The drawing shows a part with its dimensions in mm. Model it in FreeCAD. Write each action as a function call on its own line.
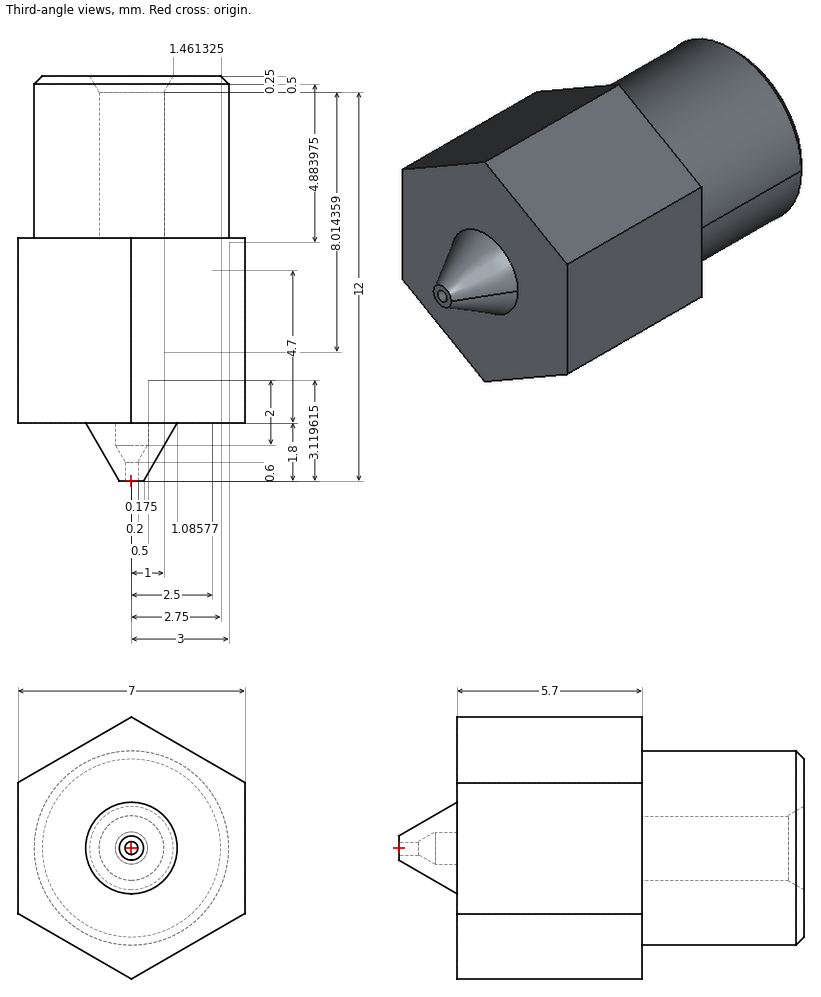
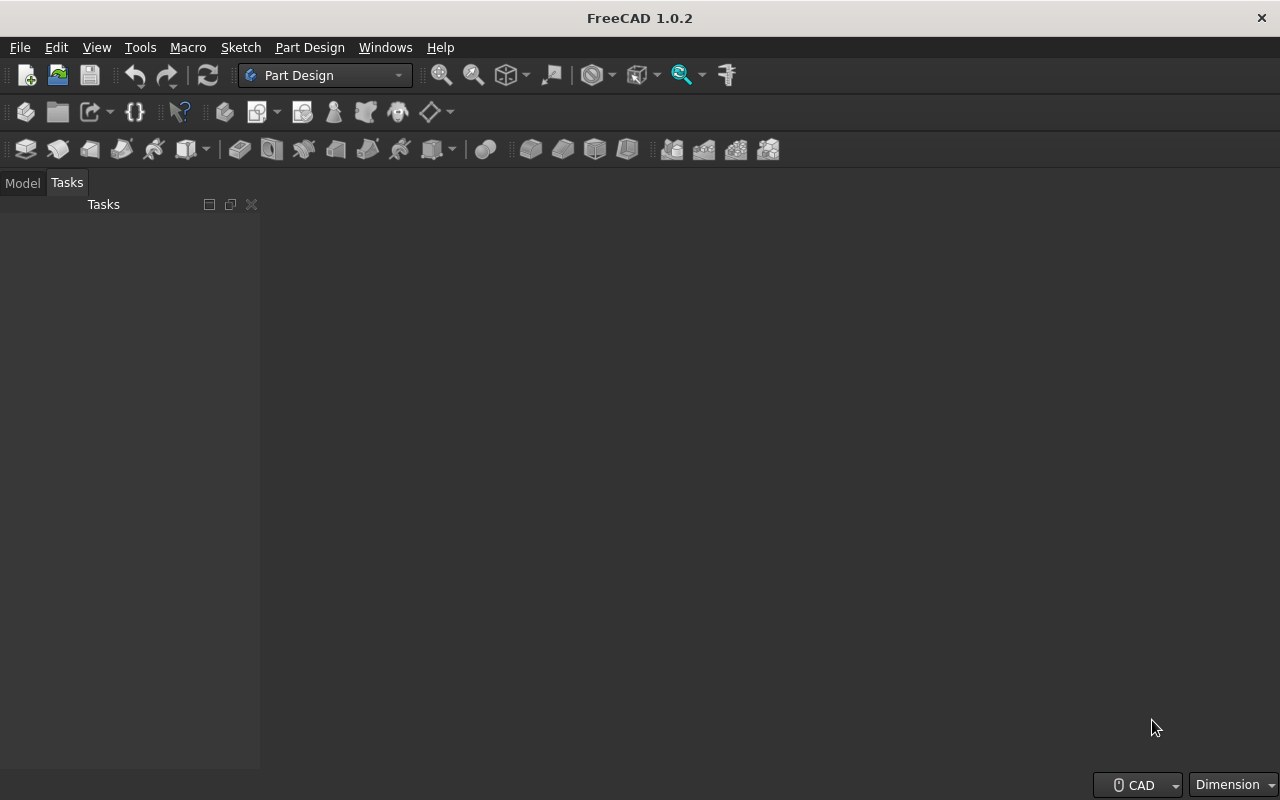
click(26, 76)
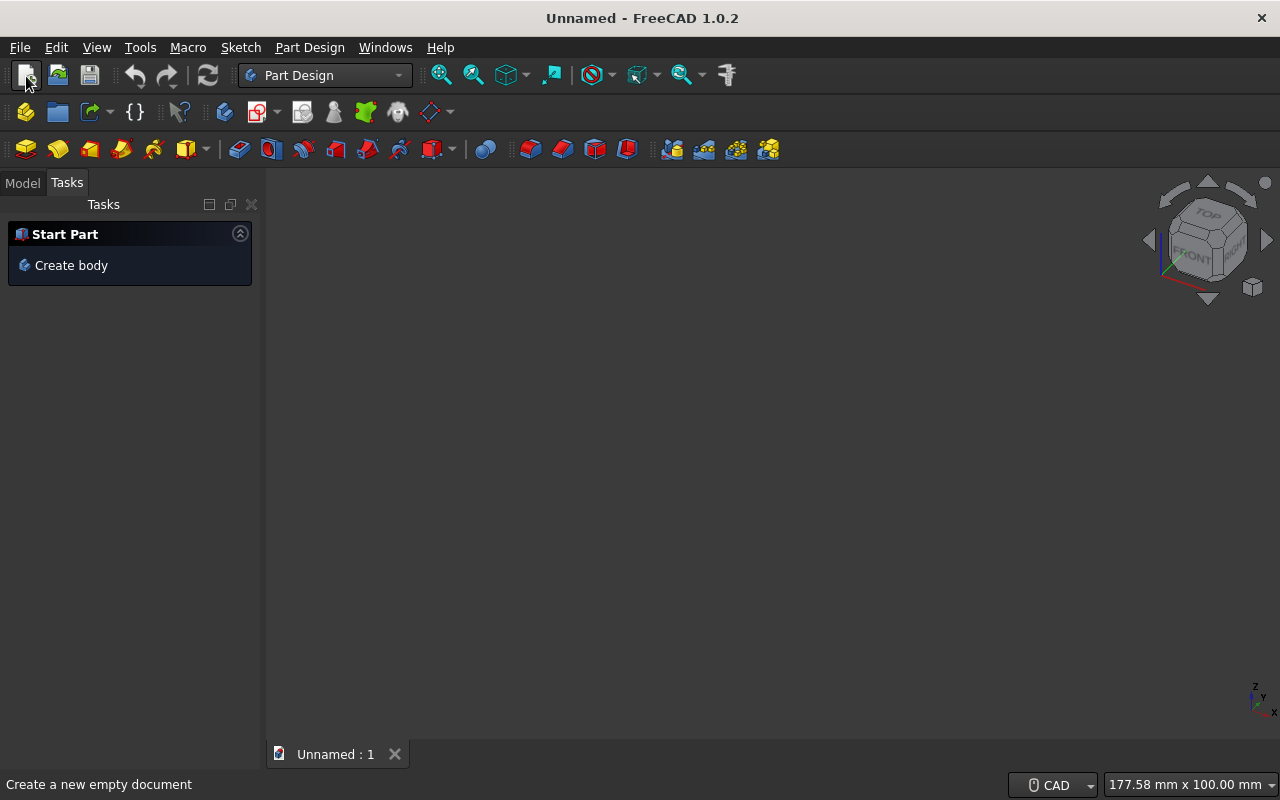
click(258, 112)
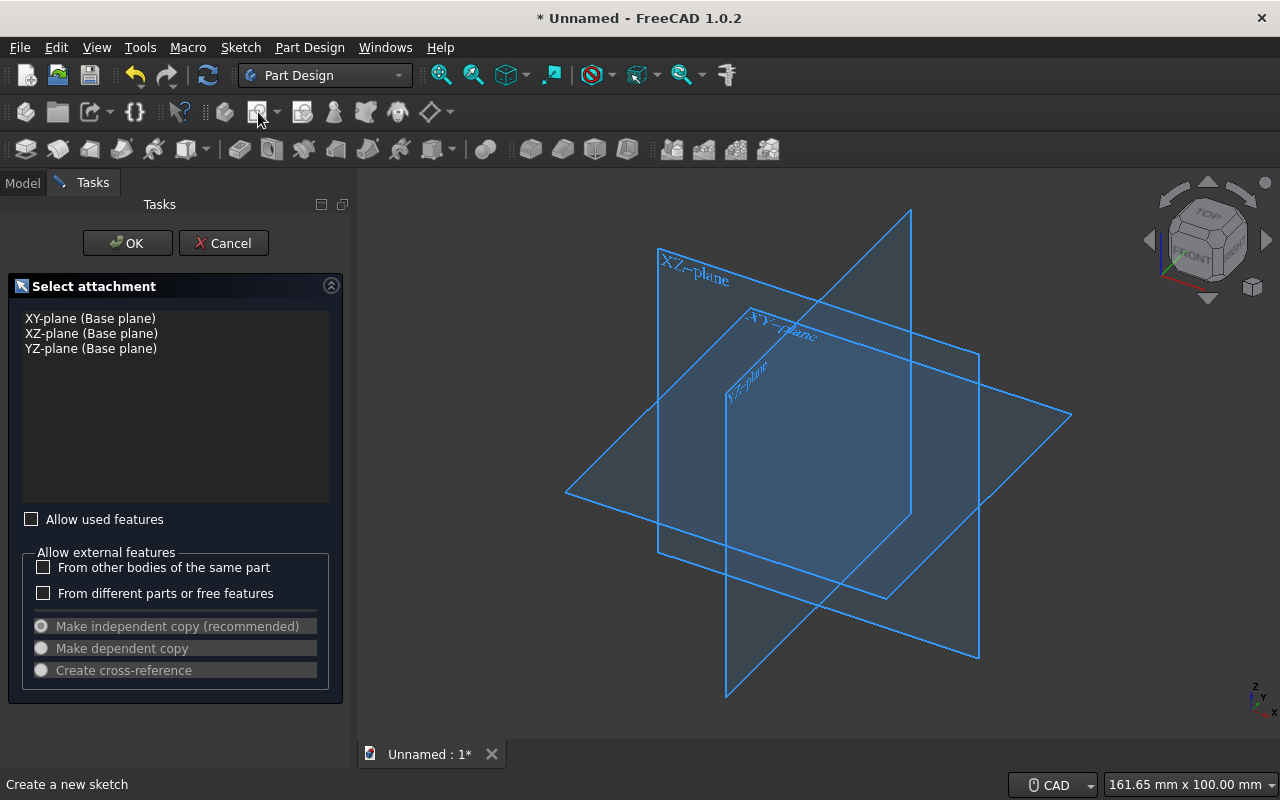
click(82, 318)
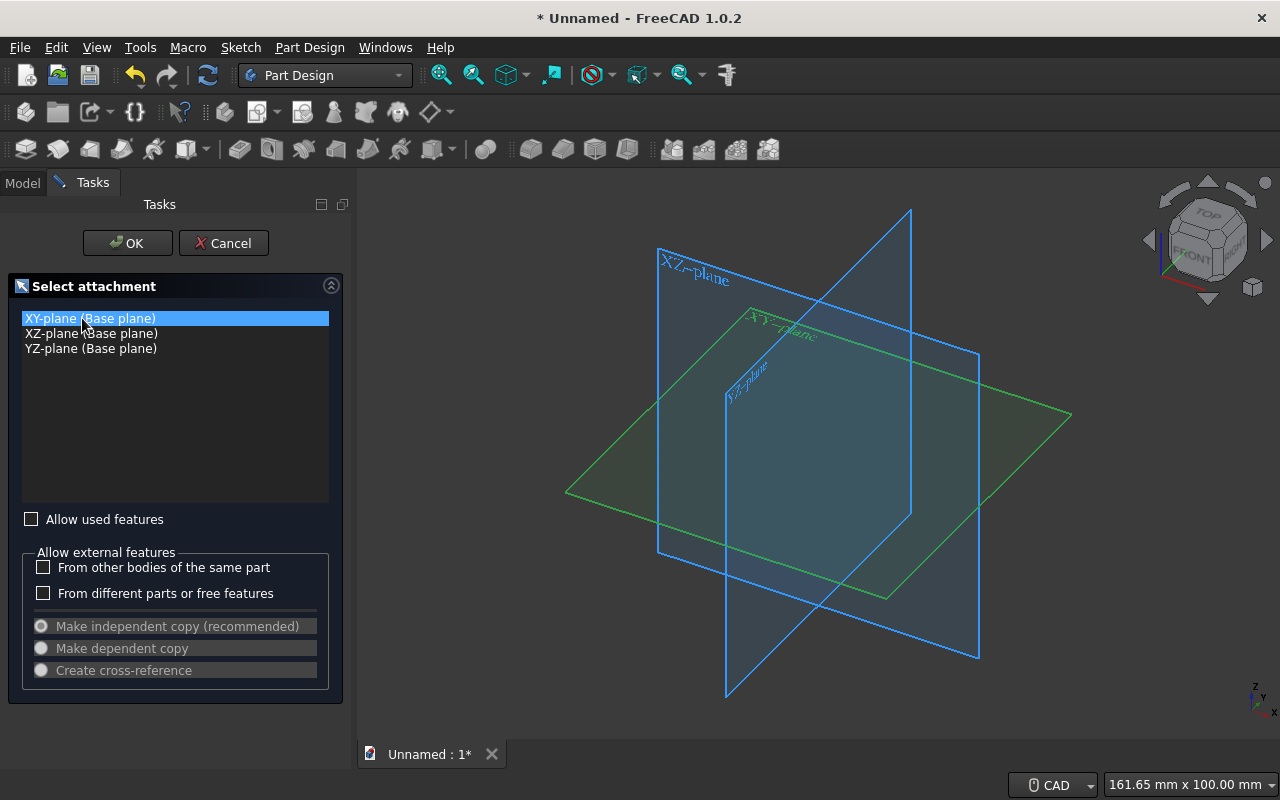
click(128, 243)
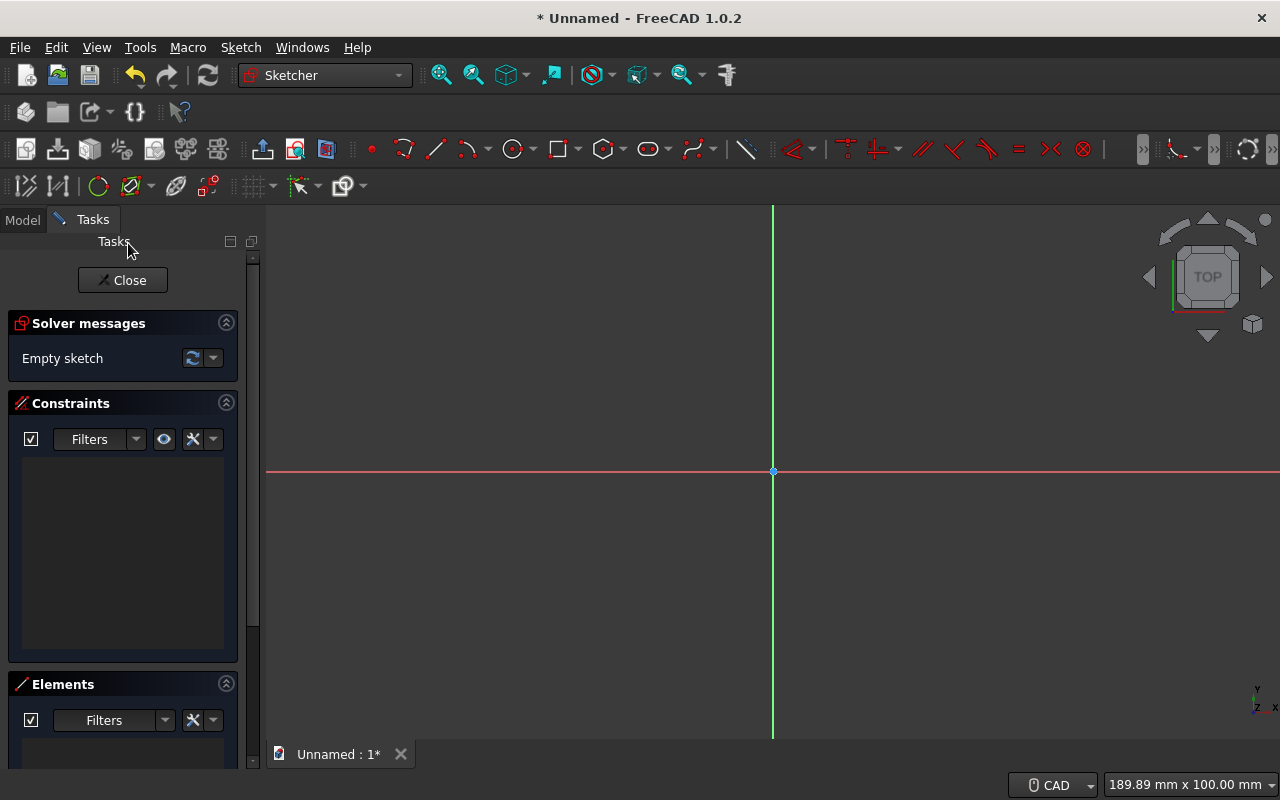
scroll(800, 430, up, 8)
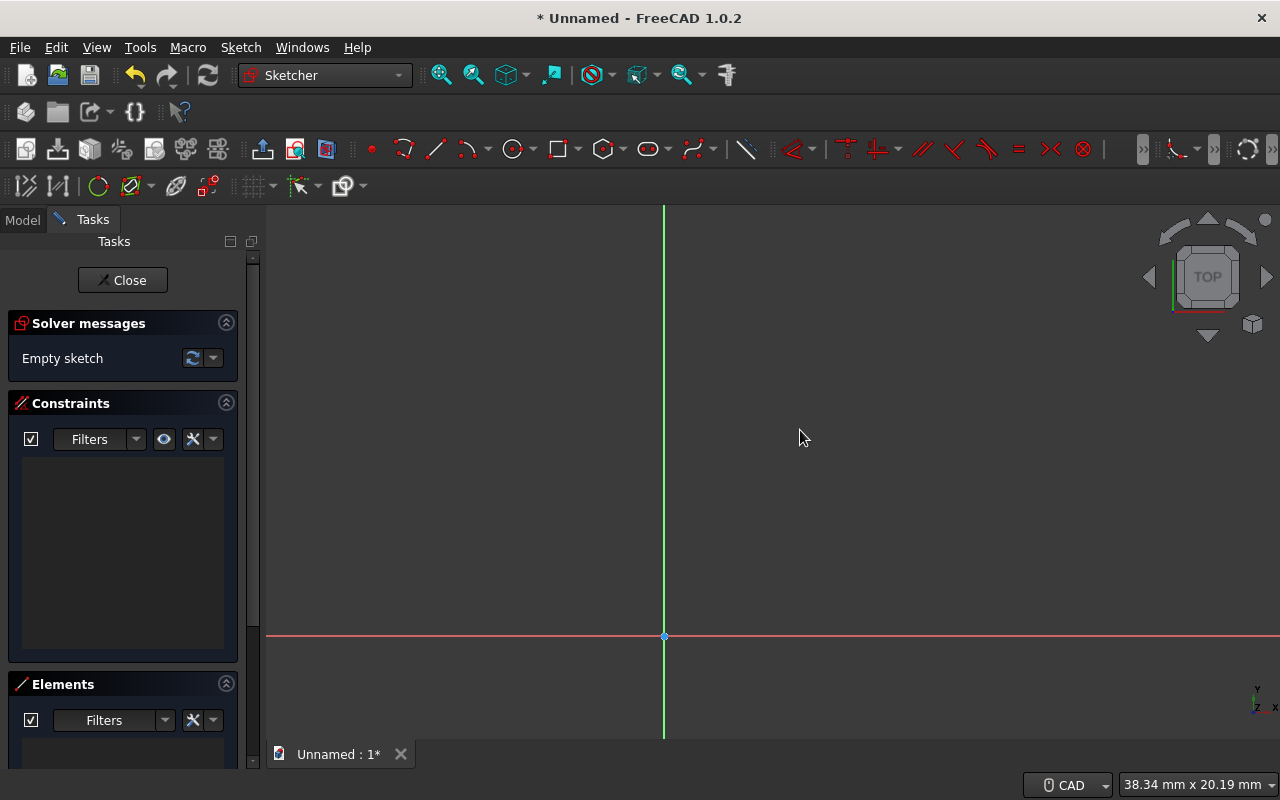
click(404, 150)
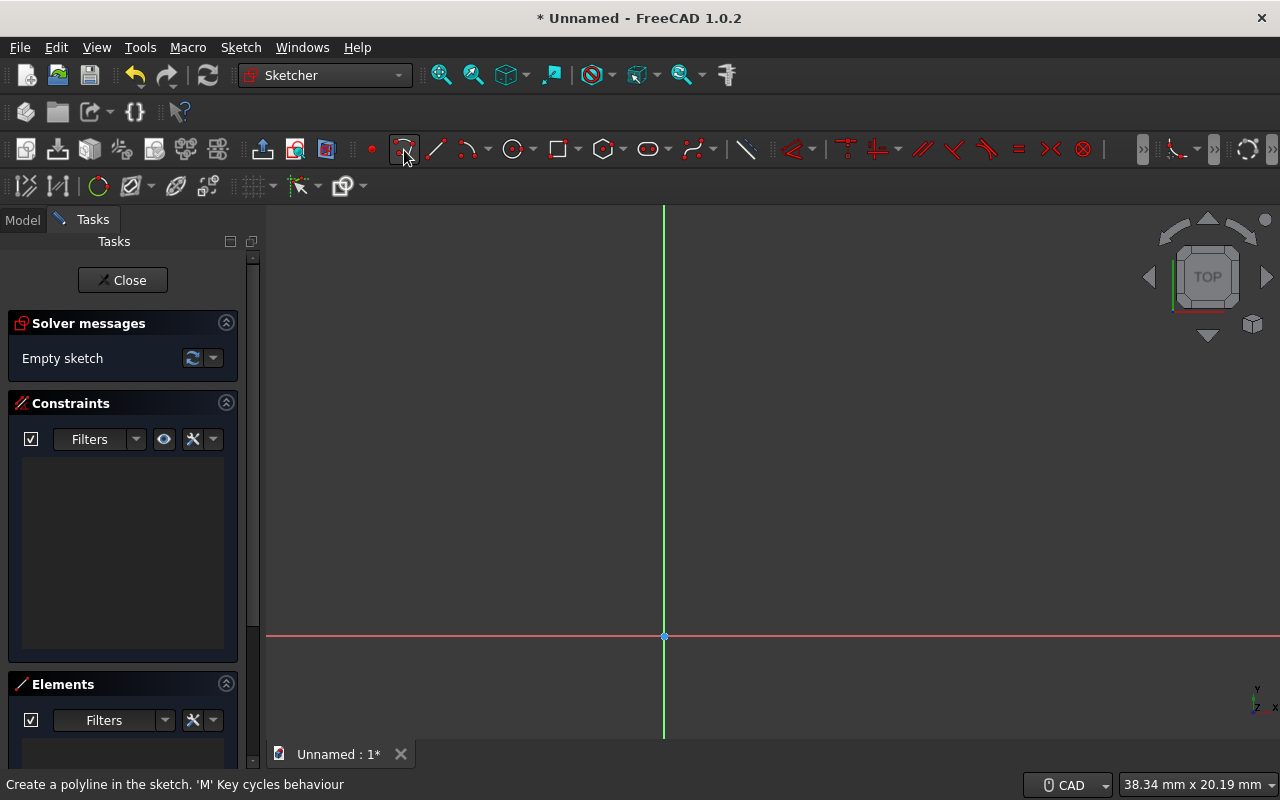
scroll(669, 636, up, 6)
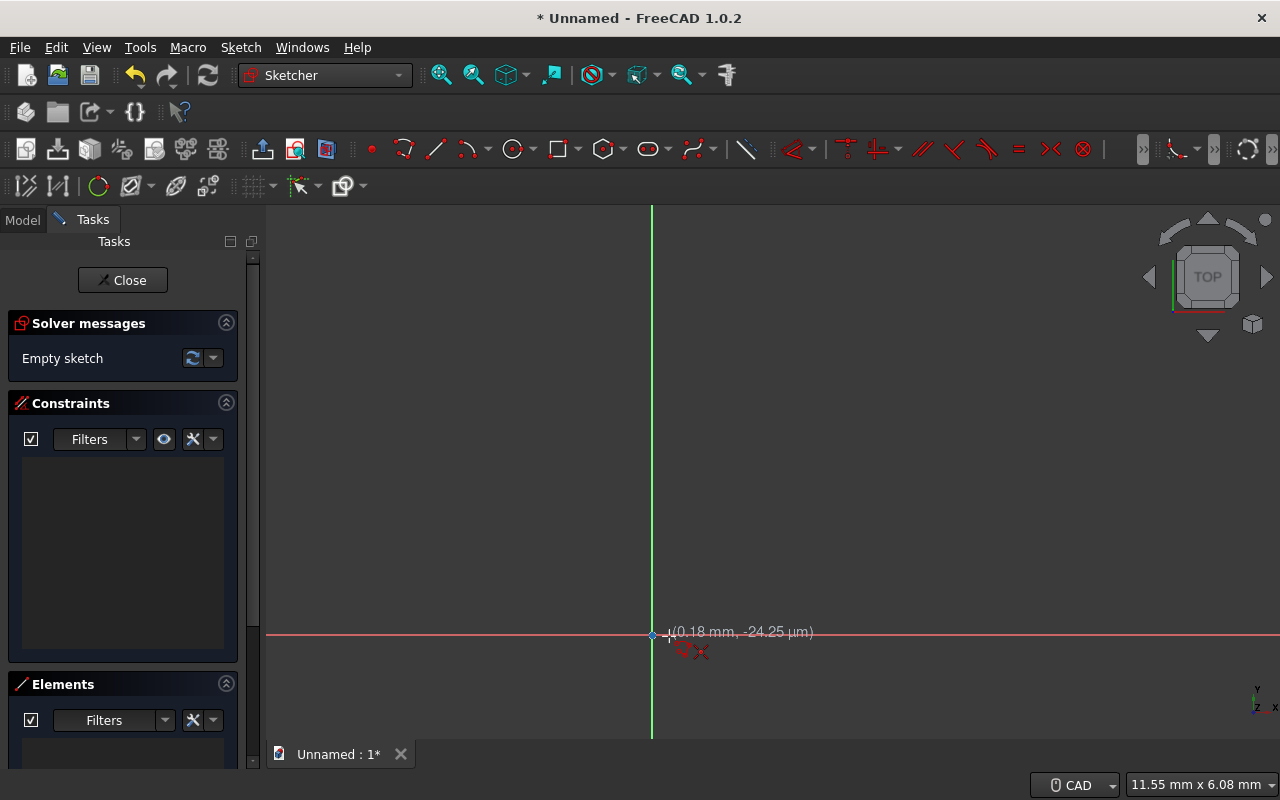
click(670, 635)
click(685, 626)
click(776, 477)
click(872, 477)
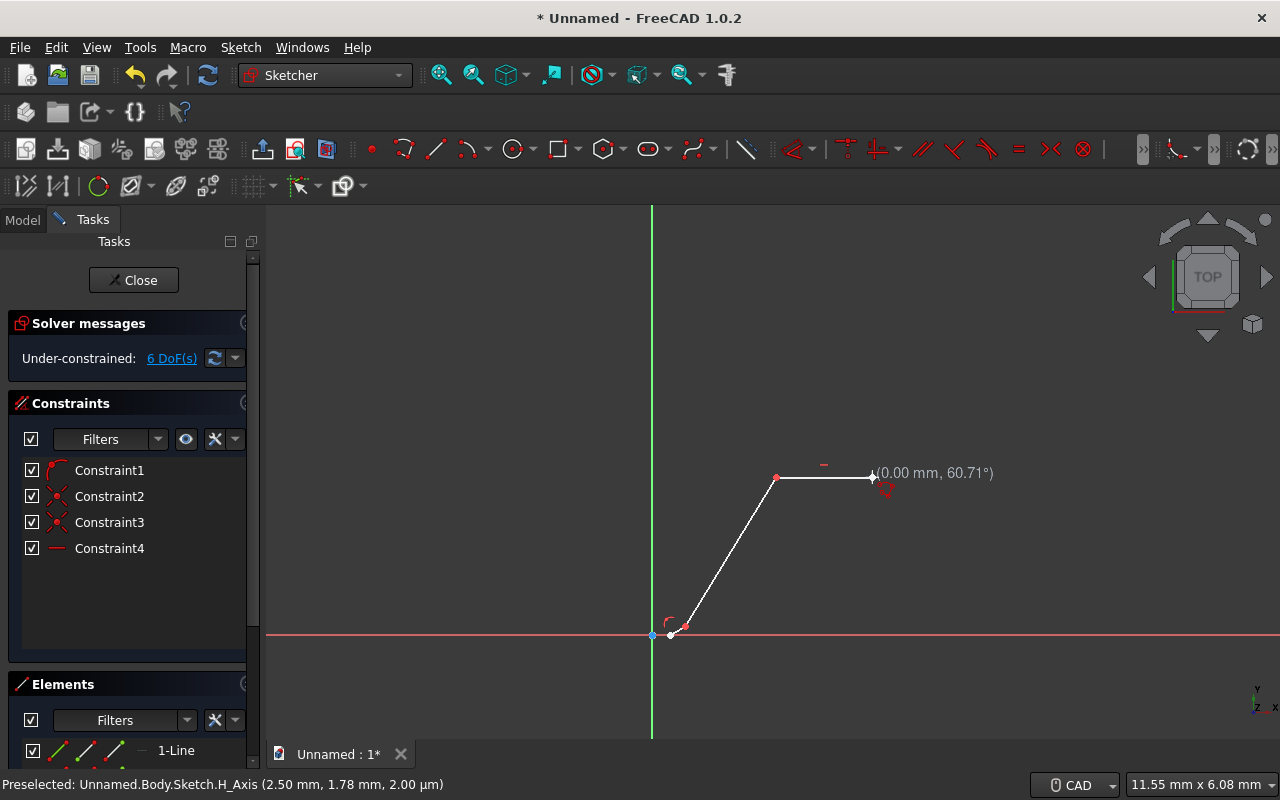
scroll(670, 638, down, 6)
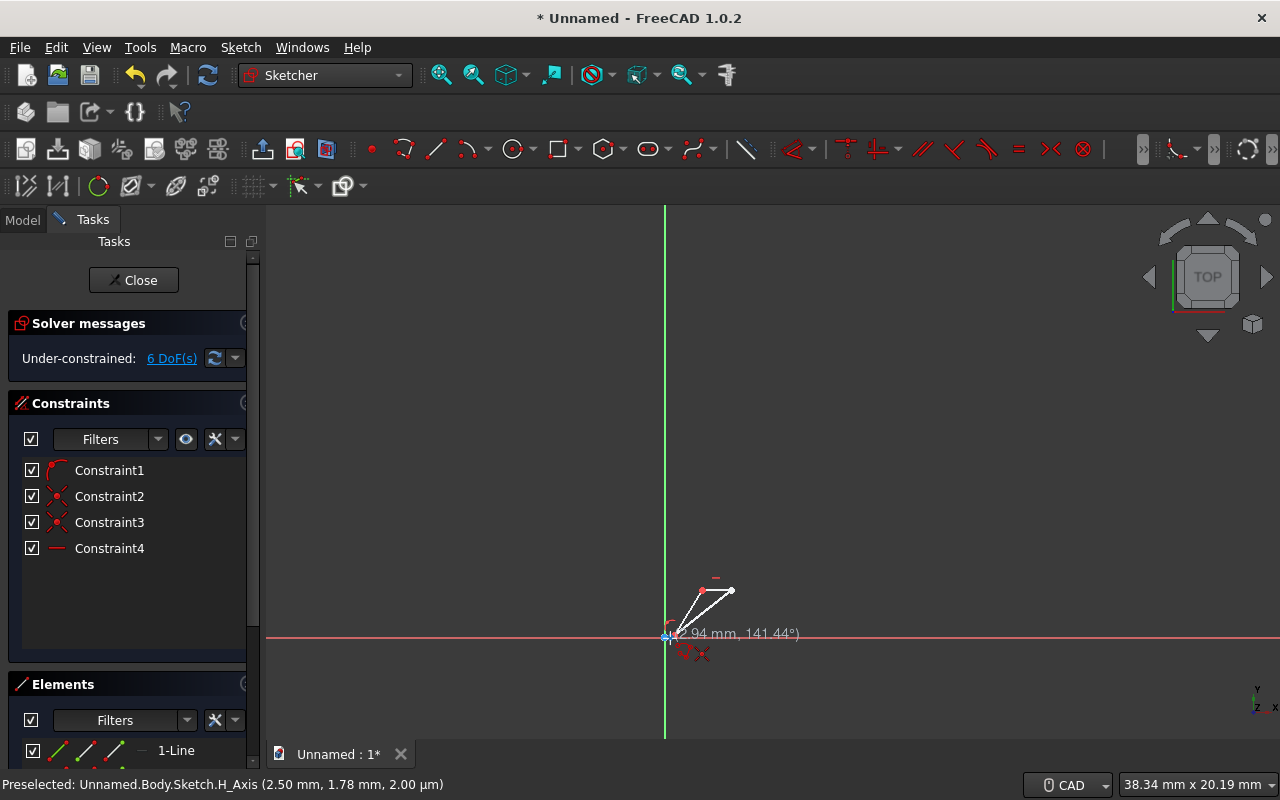
click(731, 466)
click(744, 443)
click(744, 314)